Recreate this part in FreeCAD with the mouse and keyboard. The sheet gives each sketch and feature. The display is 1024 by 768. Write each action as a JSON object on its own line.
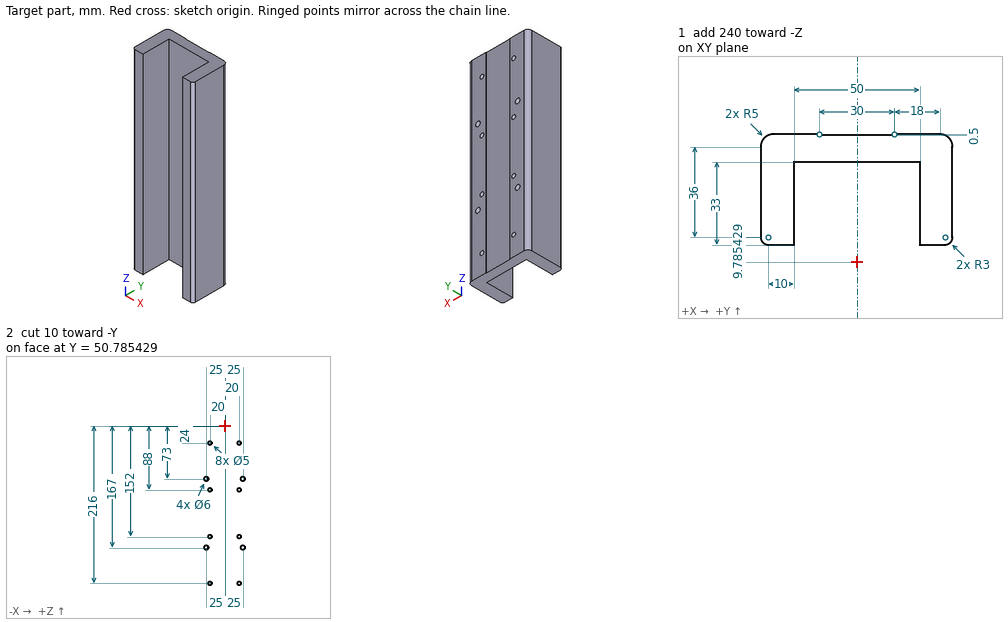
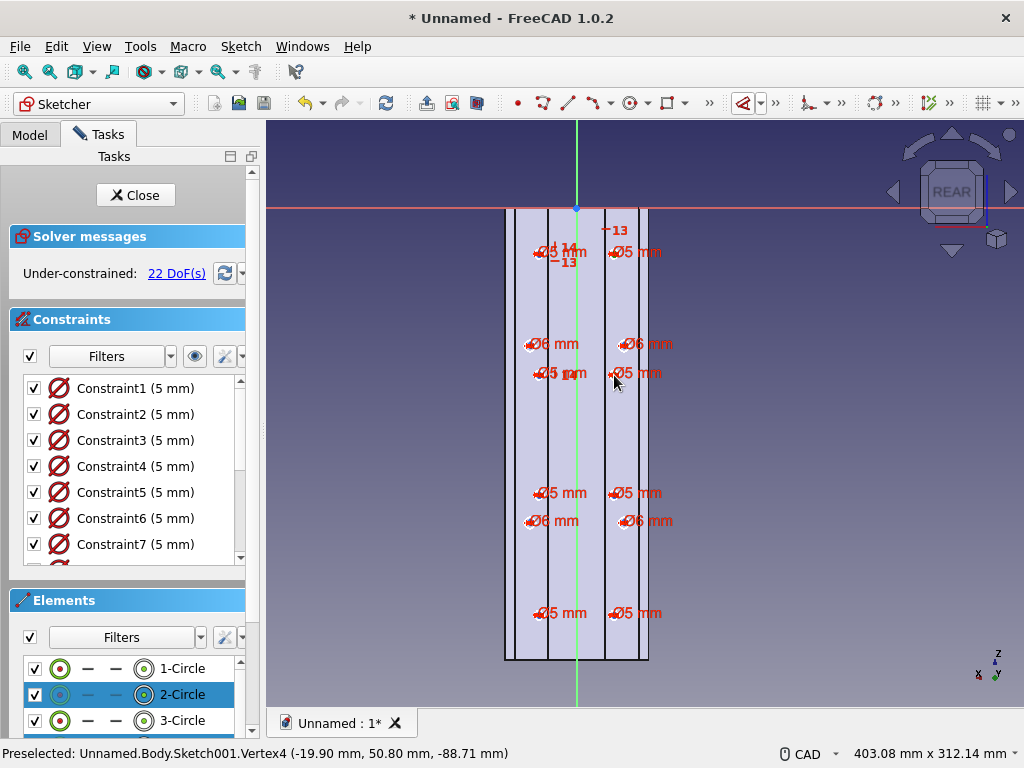
{"action": "key", "text": "v"}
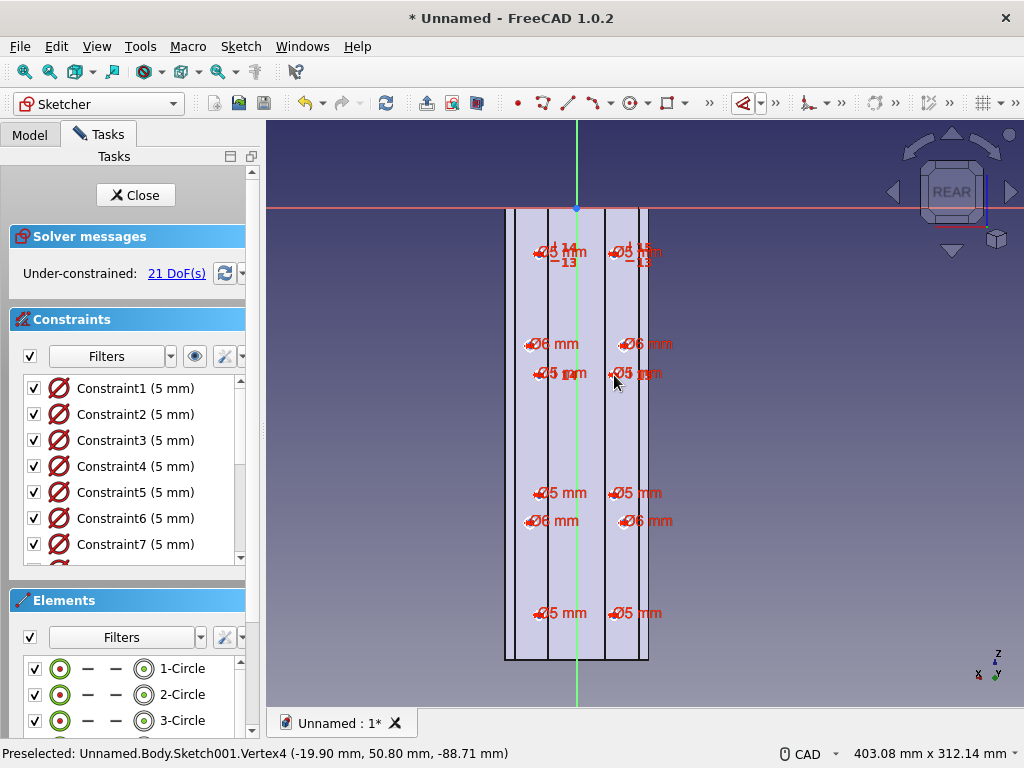
{"action": "left_click", "coordinate": [539, 375]}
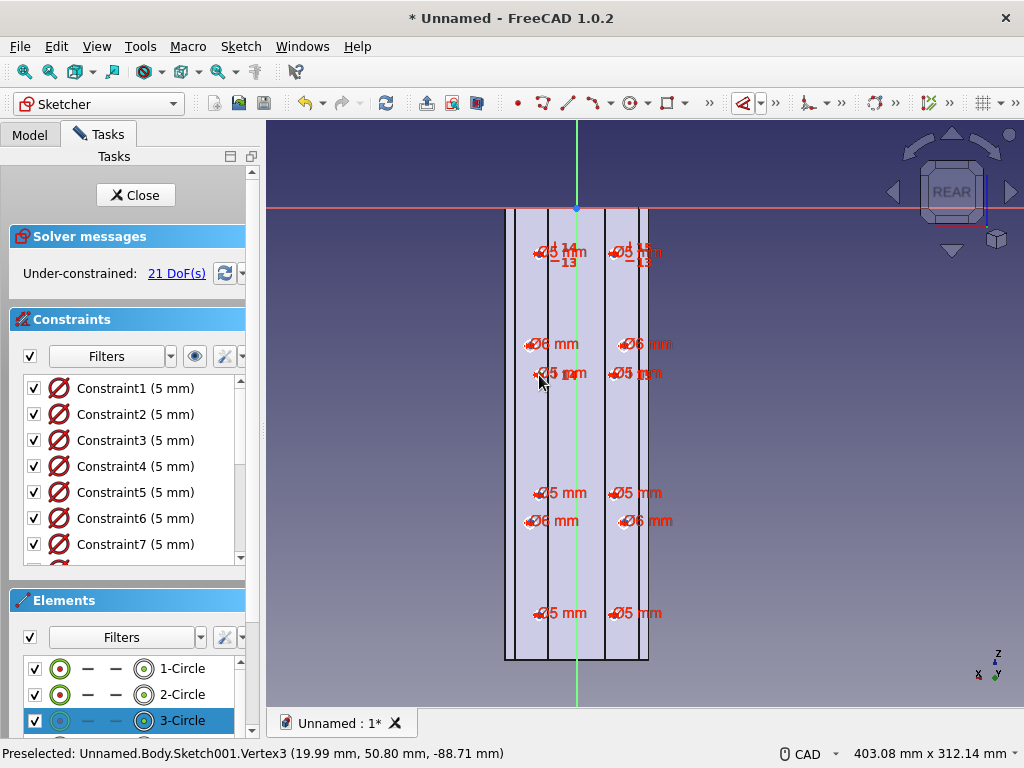
{"action": "left_click", "coordinate": [614, 375]}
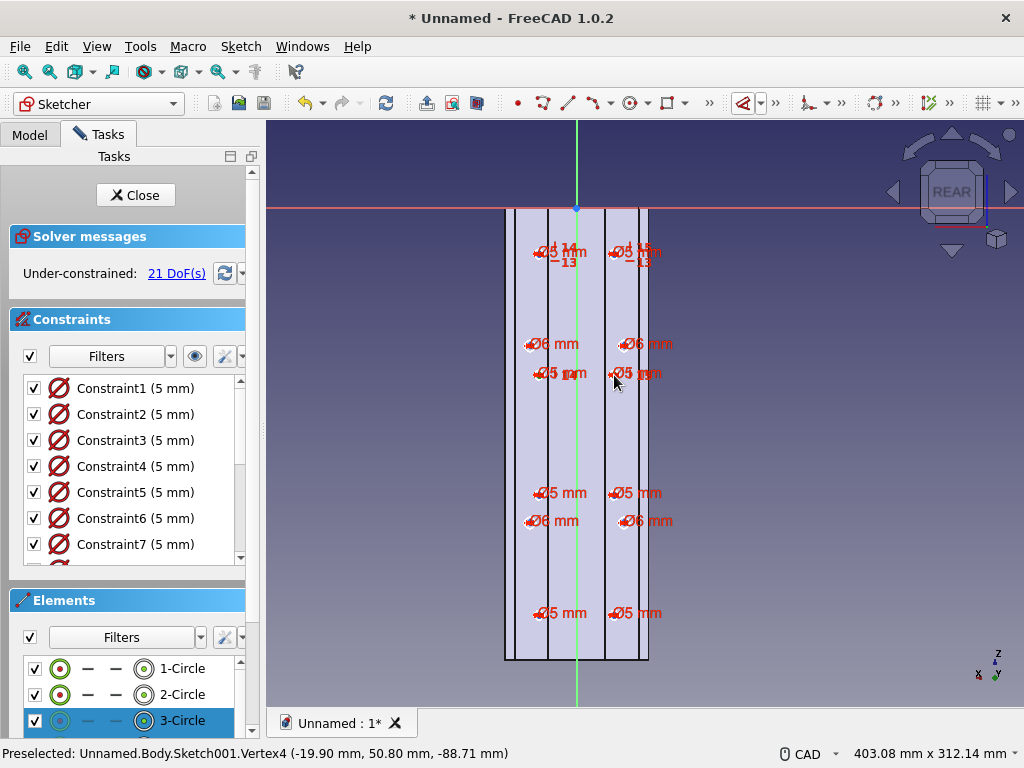
{"action": "key", "text": "h"}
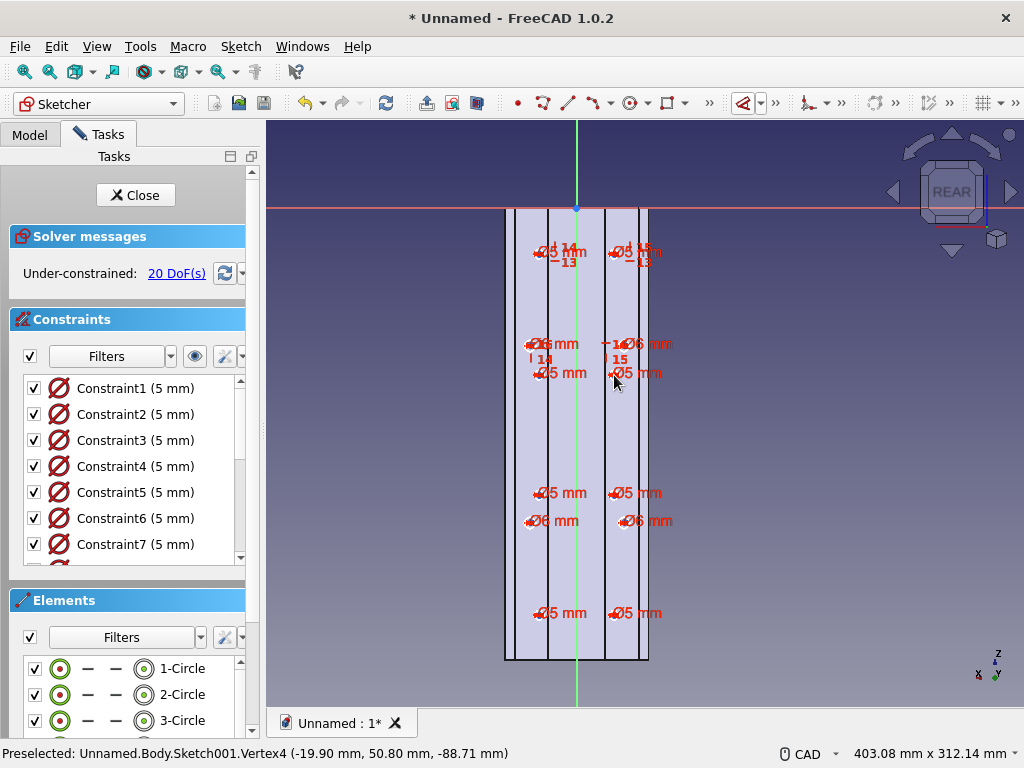
{"action": "left_click", "coordinate": [539, 375]}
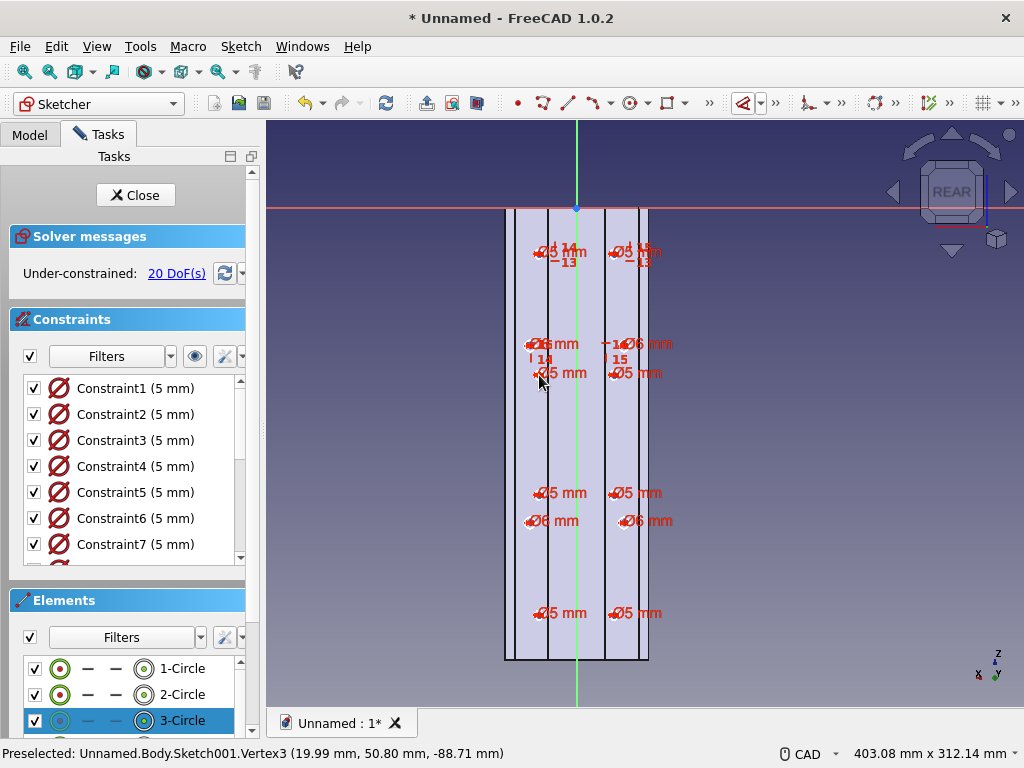
{"action": "left_click", "coordinate": [539, 495]}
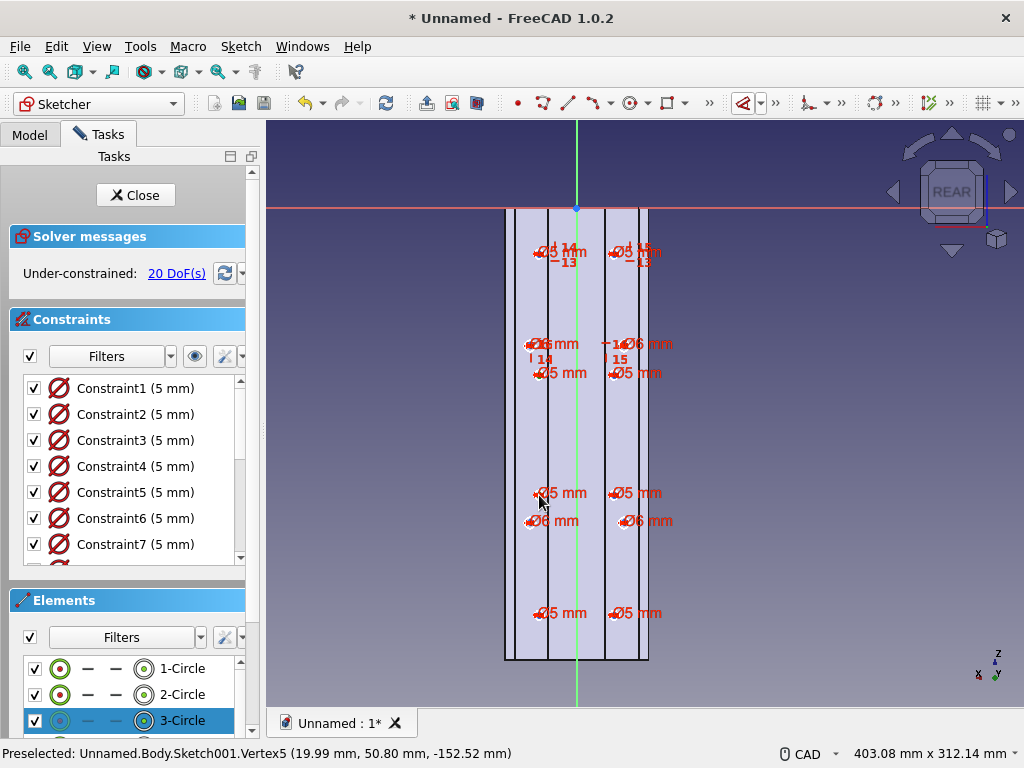
{"action": "key", "text": "v"}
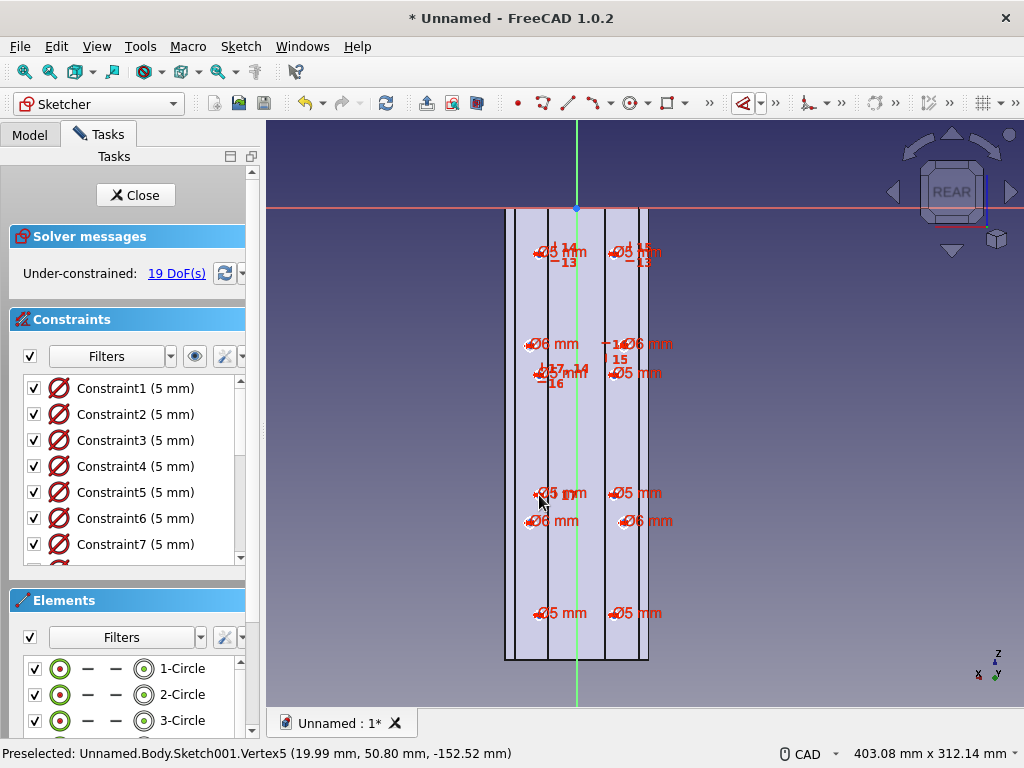
{"action": "left_click", "coordinate": [614, 375]}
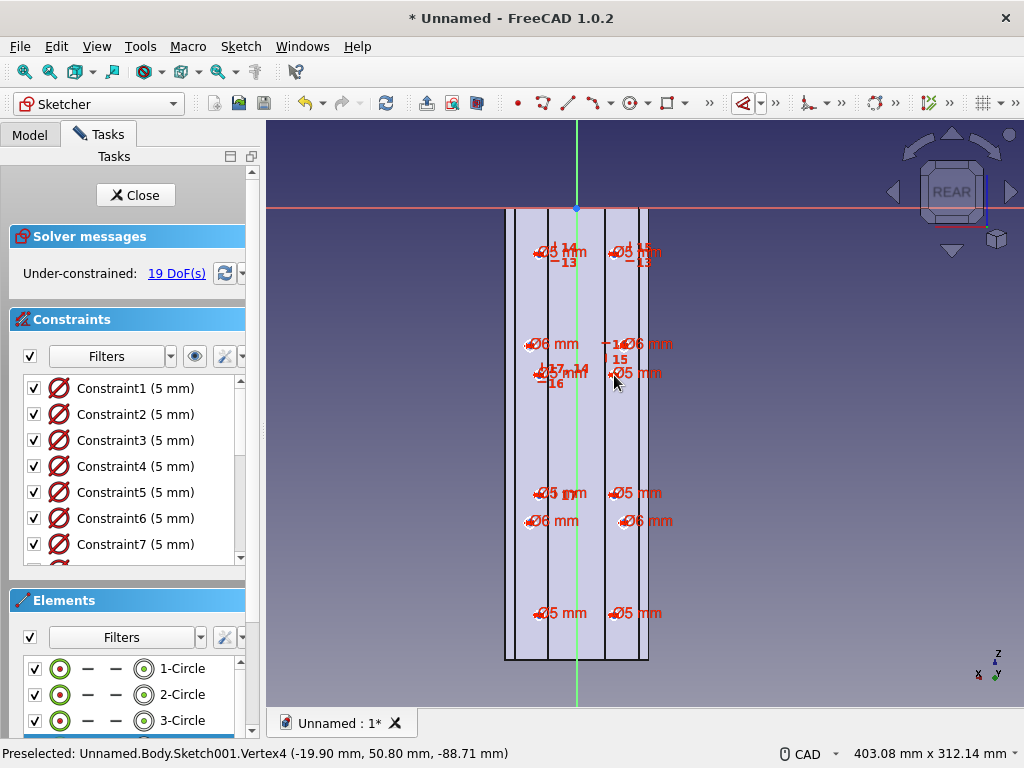
{"action": "left_click", "coordinate": [614, 495]}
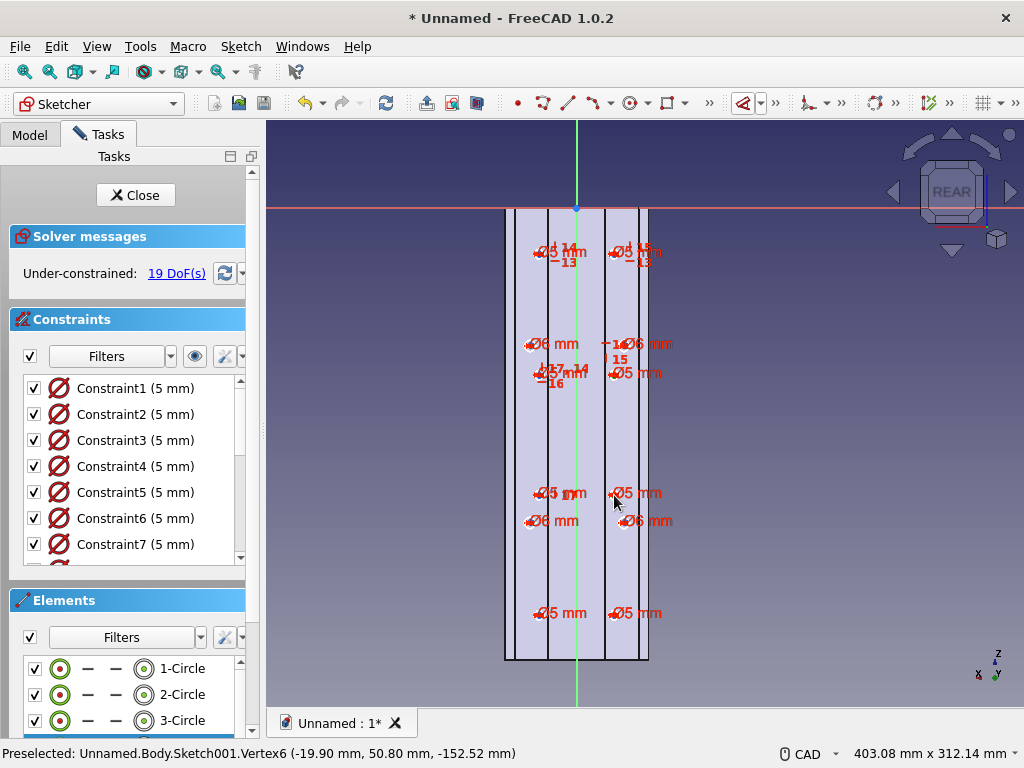
{"action": "key", "text": "v"}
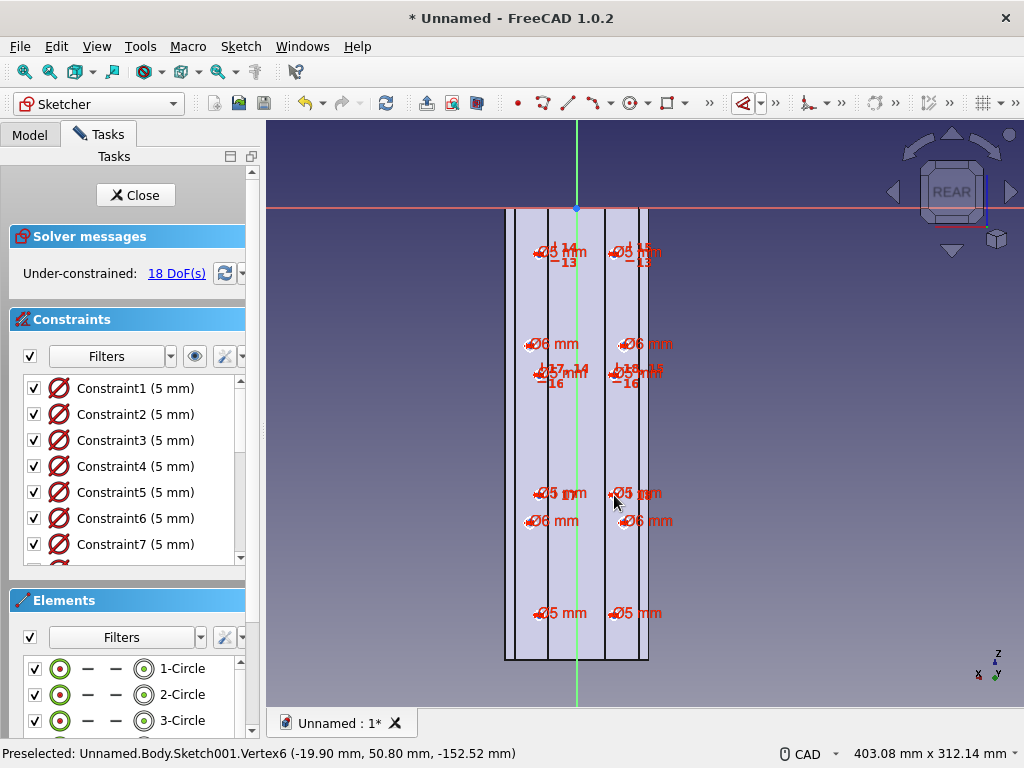
{"action": "left_click", "coordinate": [539, 495]}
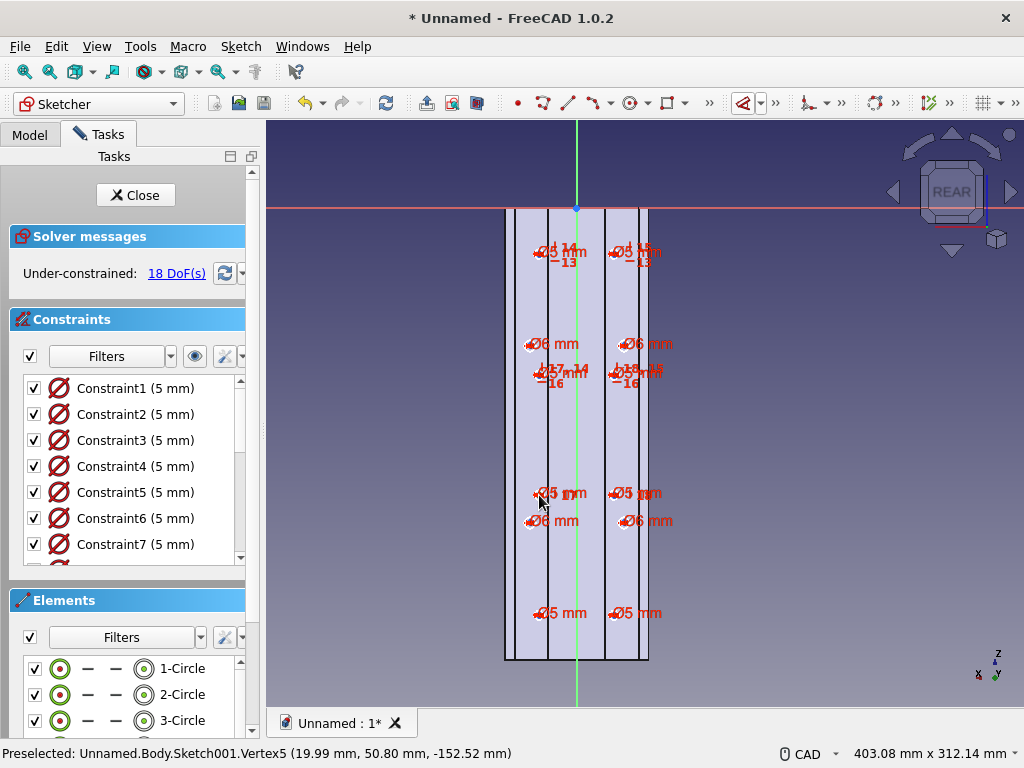
{"action": "left_click", "coordinate": [614, 495]}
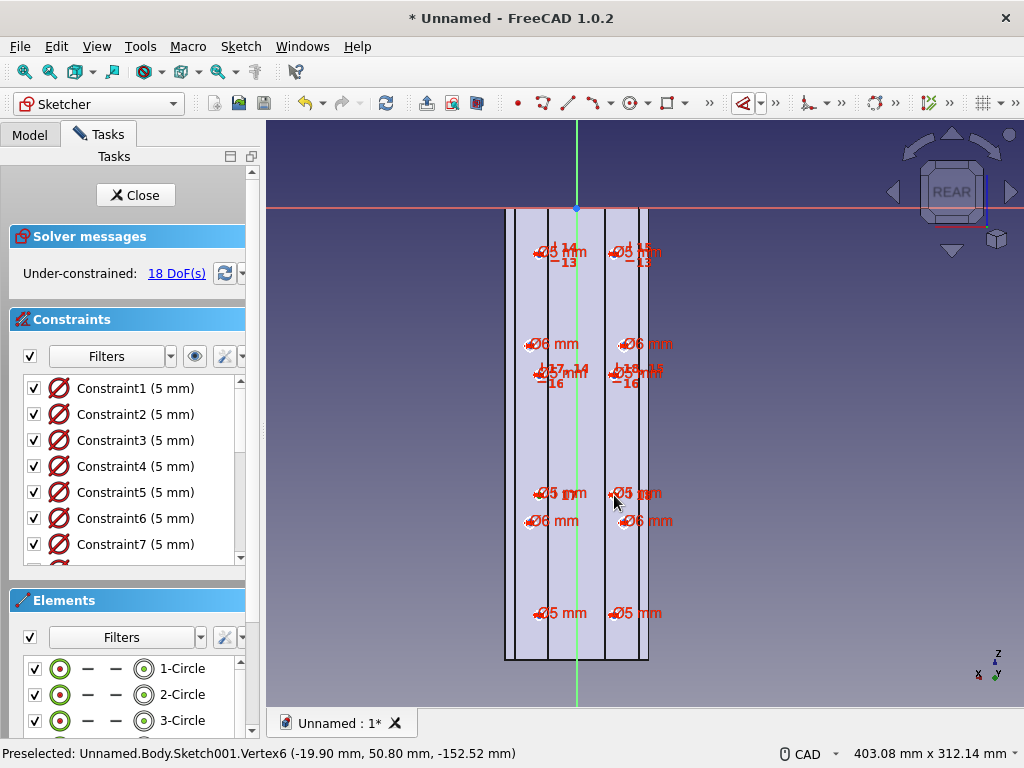
{"action": "key", "text": "h"}